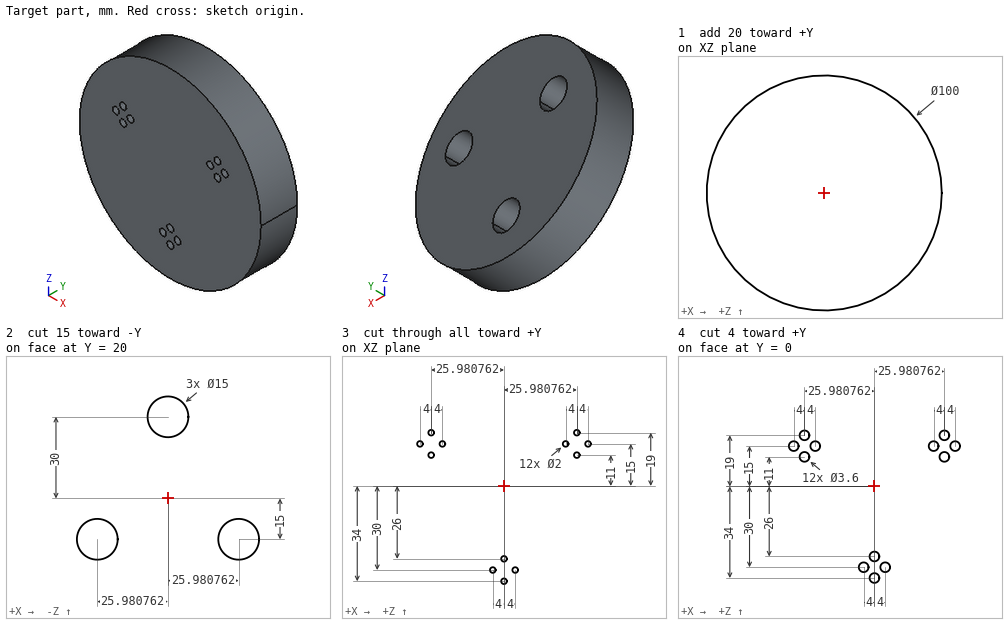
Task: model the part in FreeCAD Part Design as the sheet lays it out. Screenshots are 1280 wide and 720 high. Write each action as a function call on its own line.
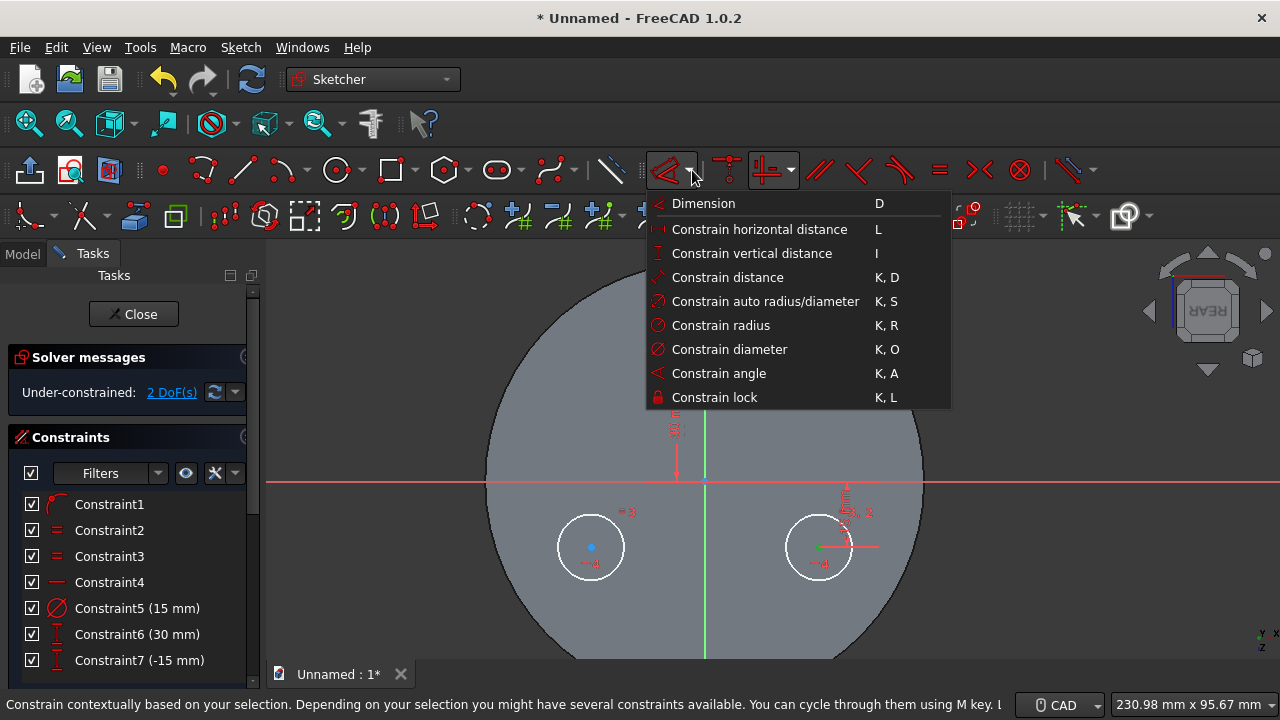
click(799, 229)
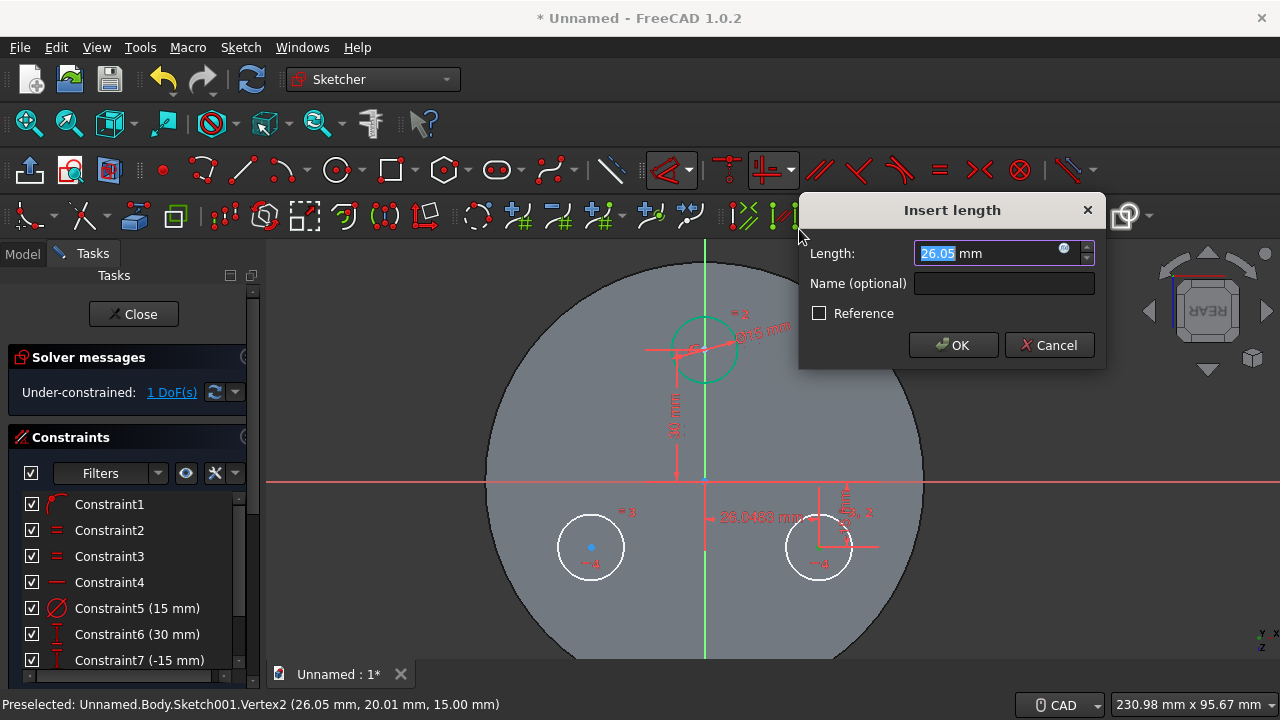
text(25.980762)
key(Return)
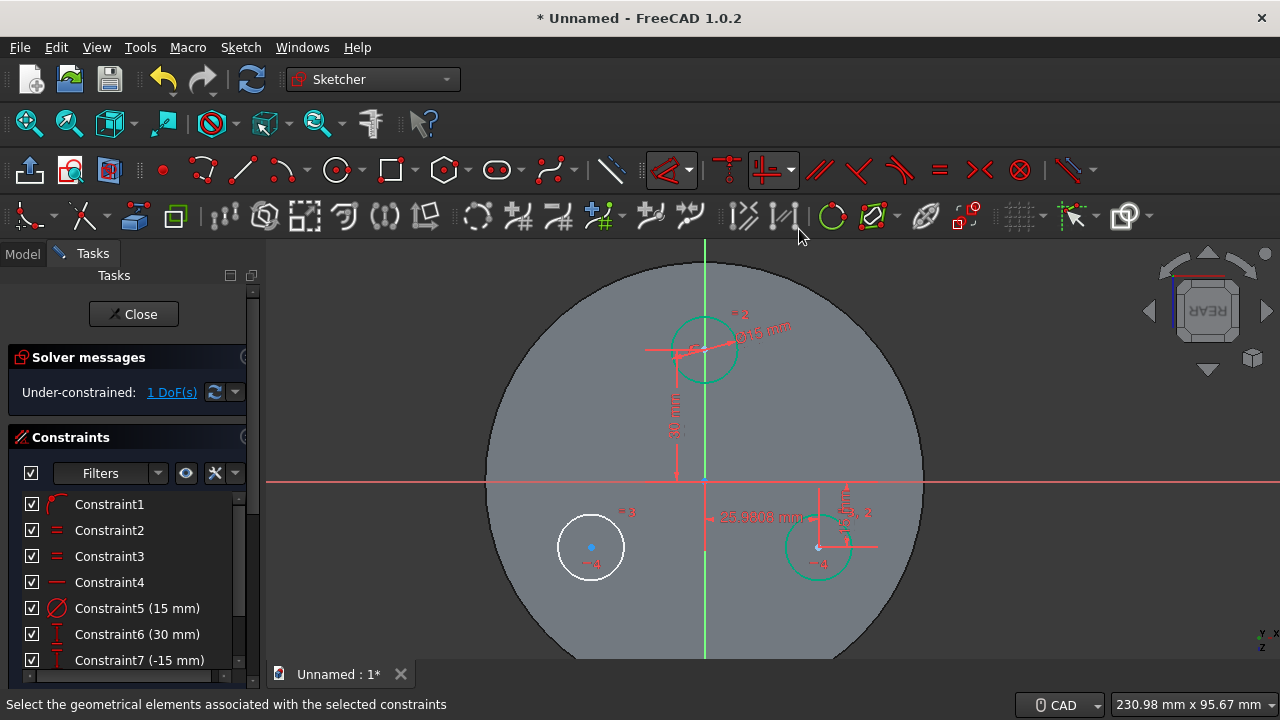
click(591, 547)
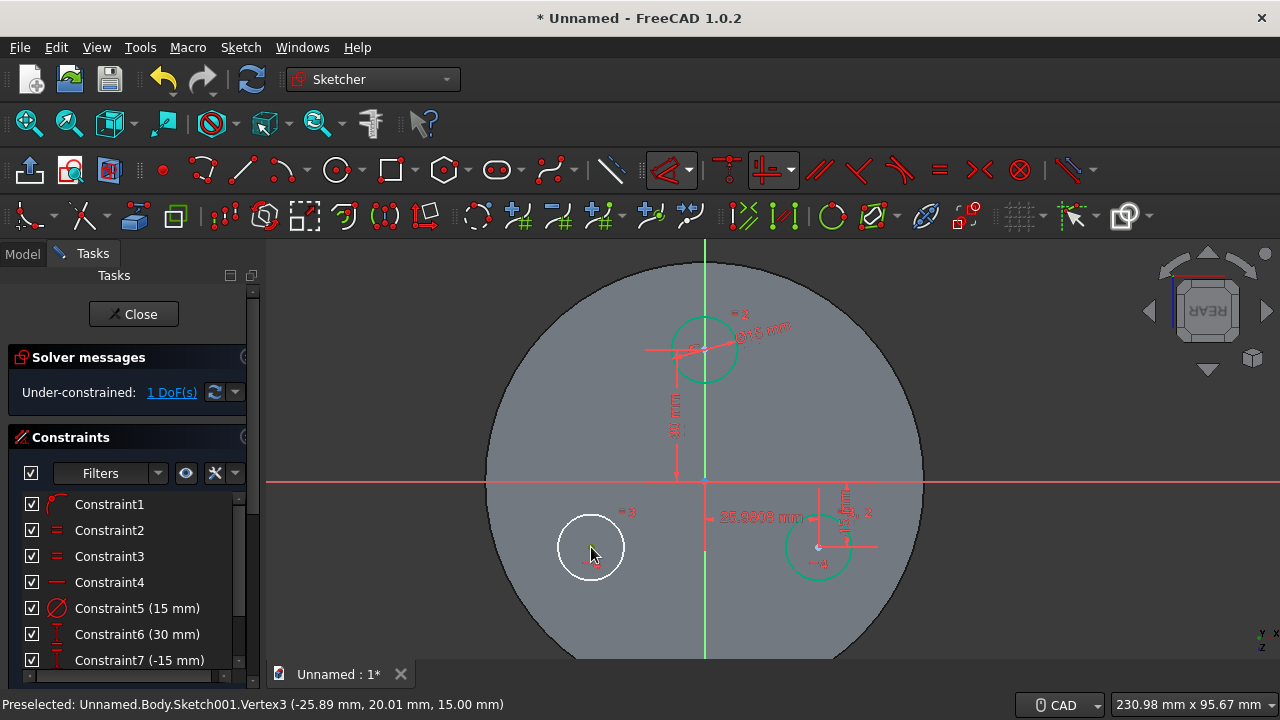
click(692, 170)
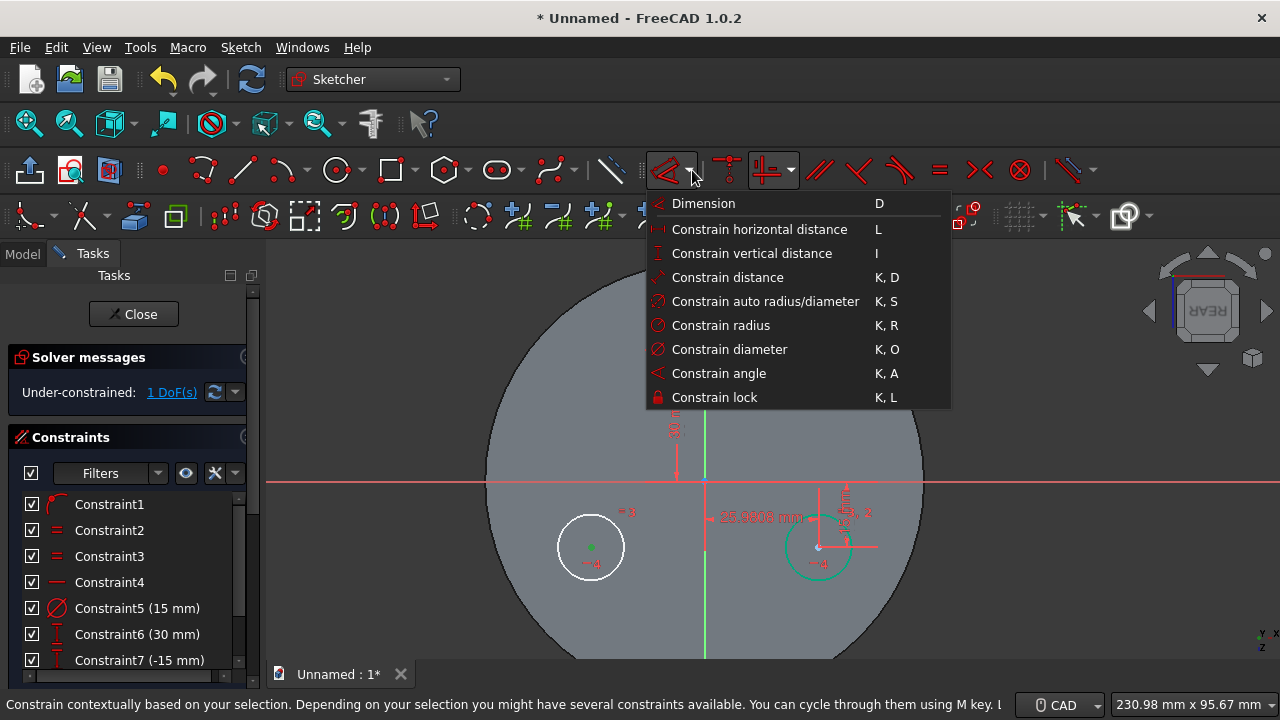
click(799, 229)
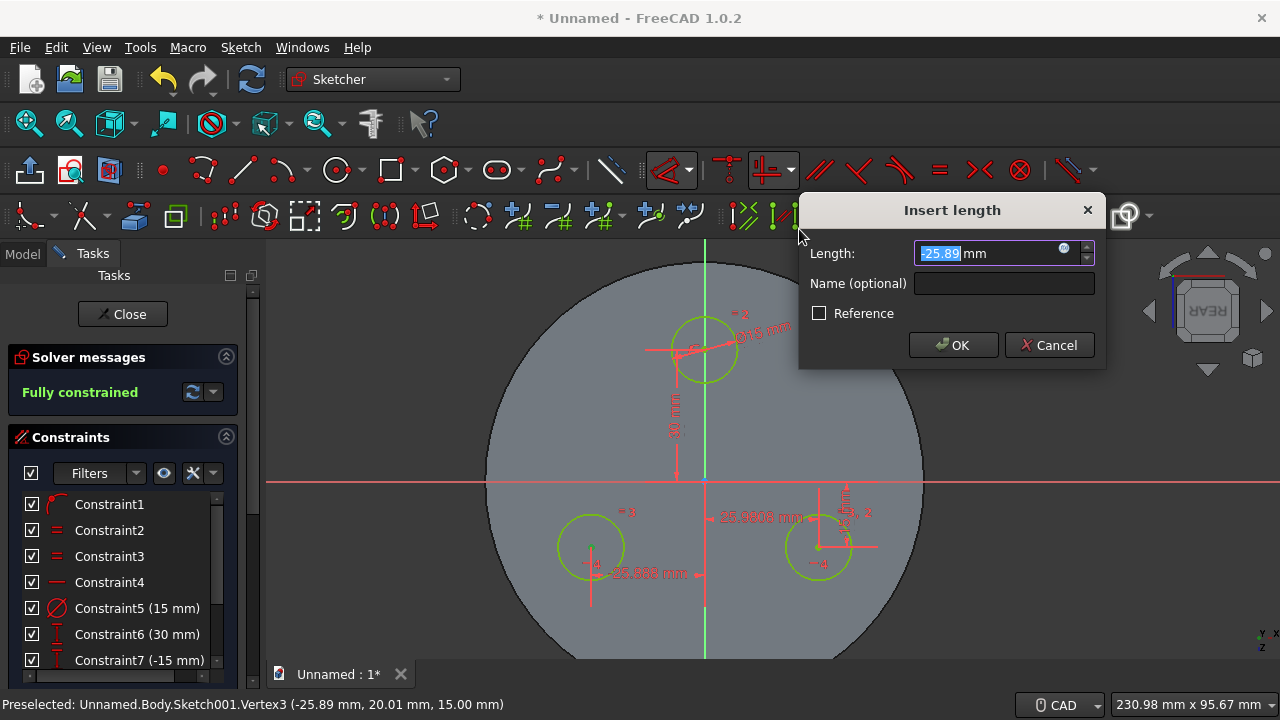
text(-25.980762)
key(Return)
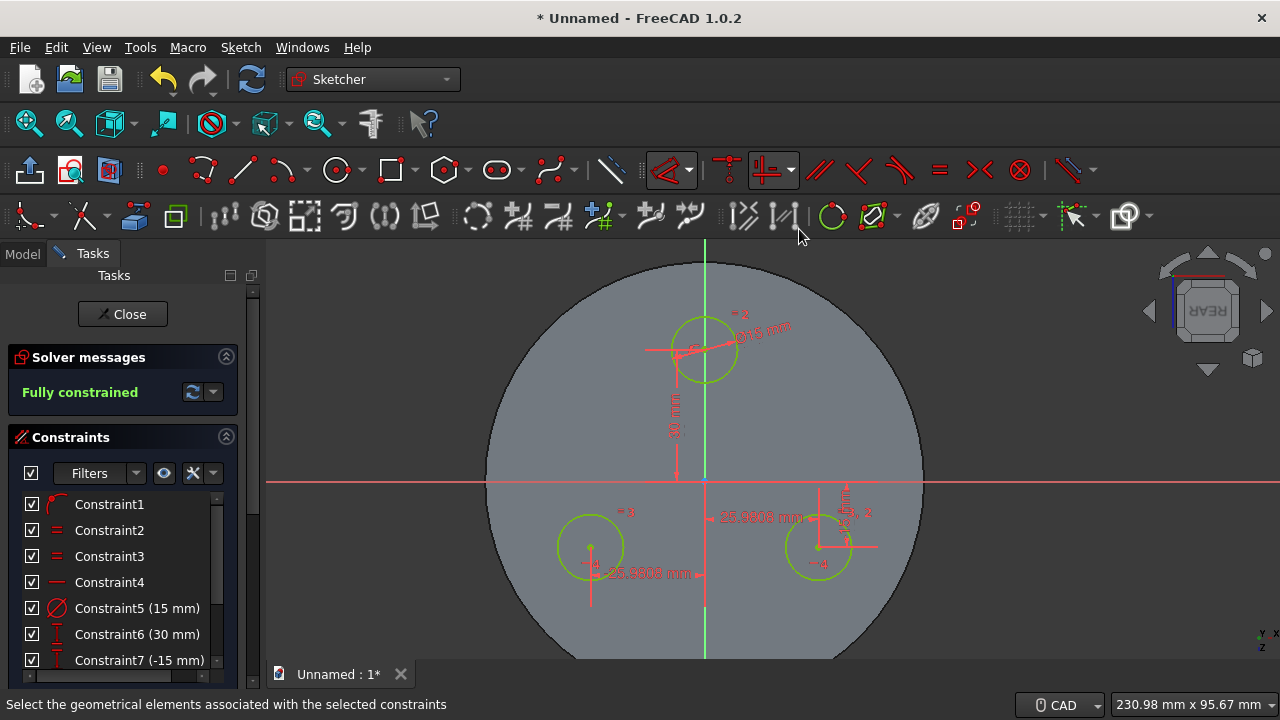
click(123, 314)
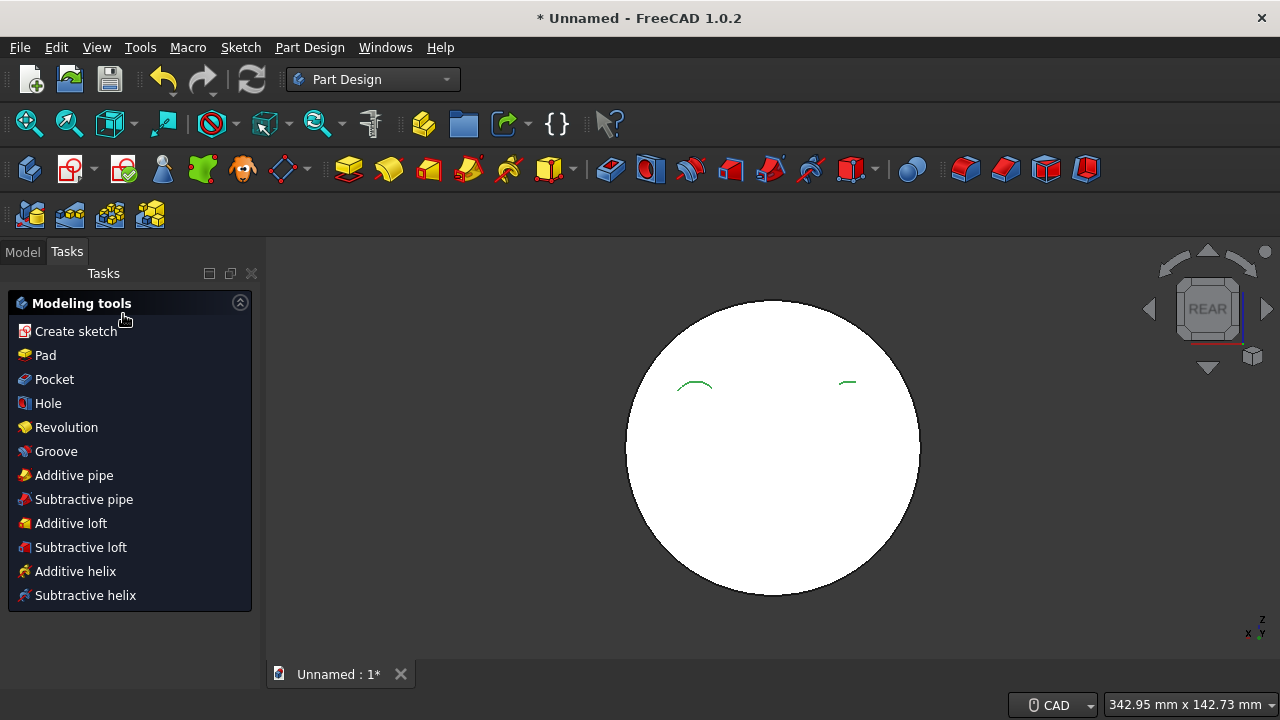
click(612, 170)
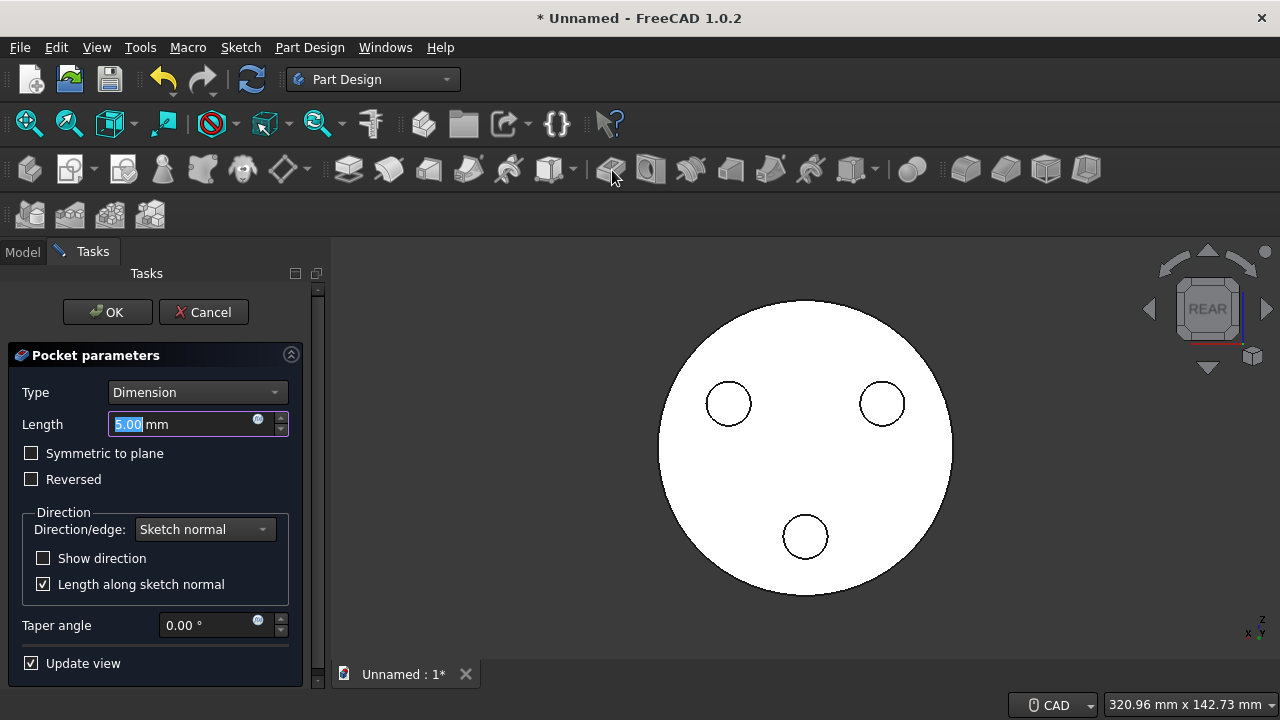
text(15)
key(Tab)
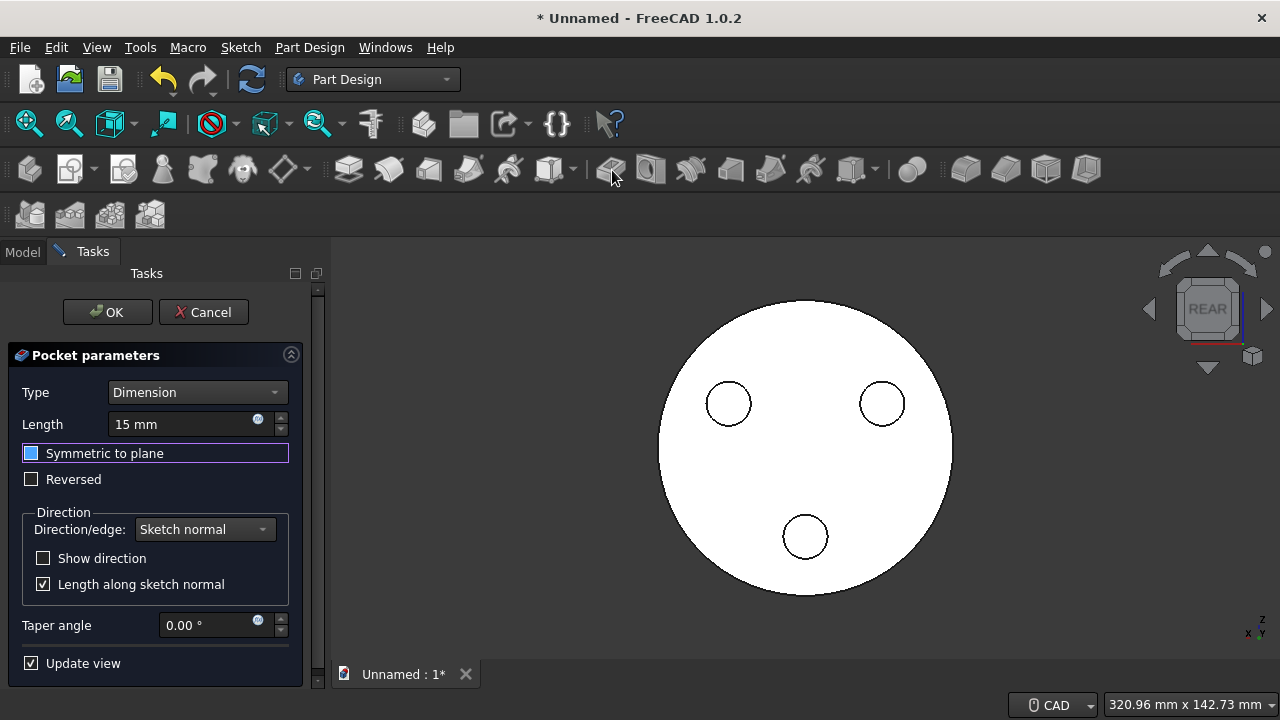
click(108, 312)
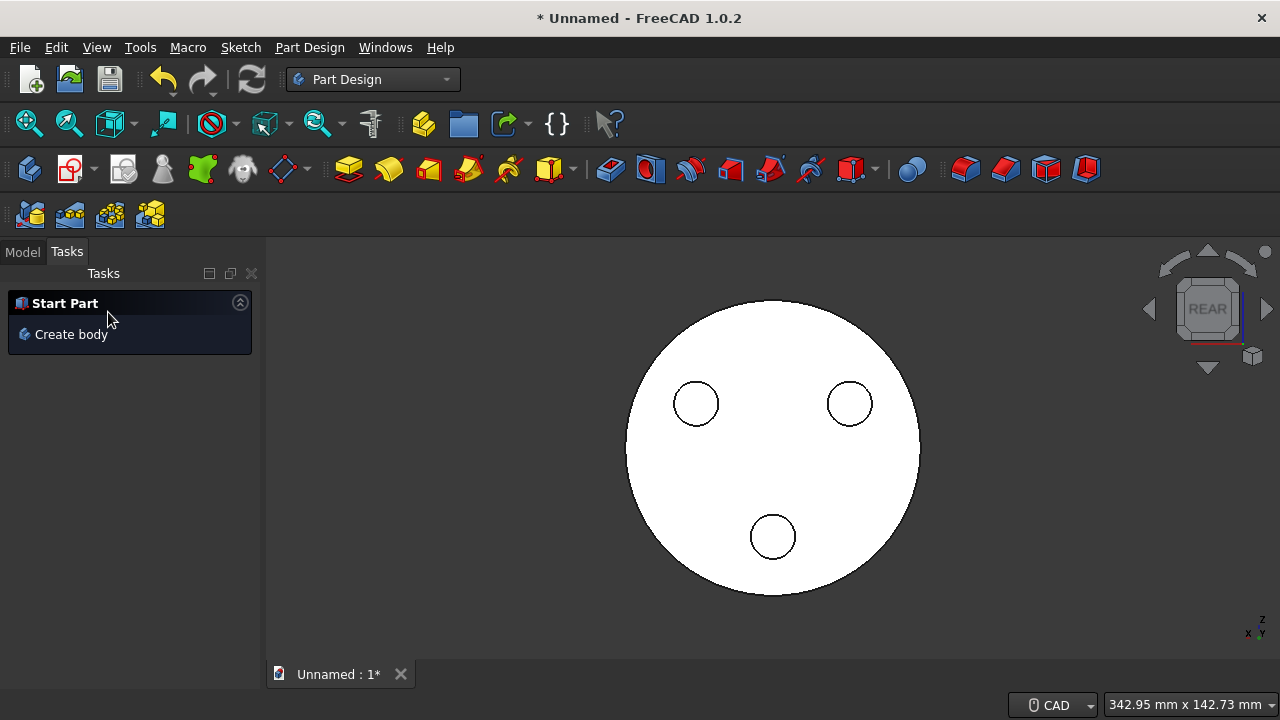
click(70, 170)